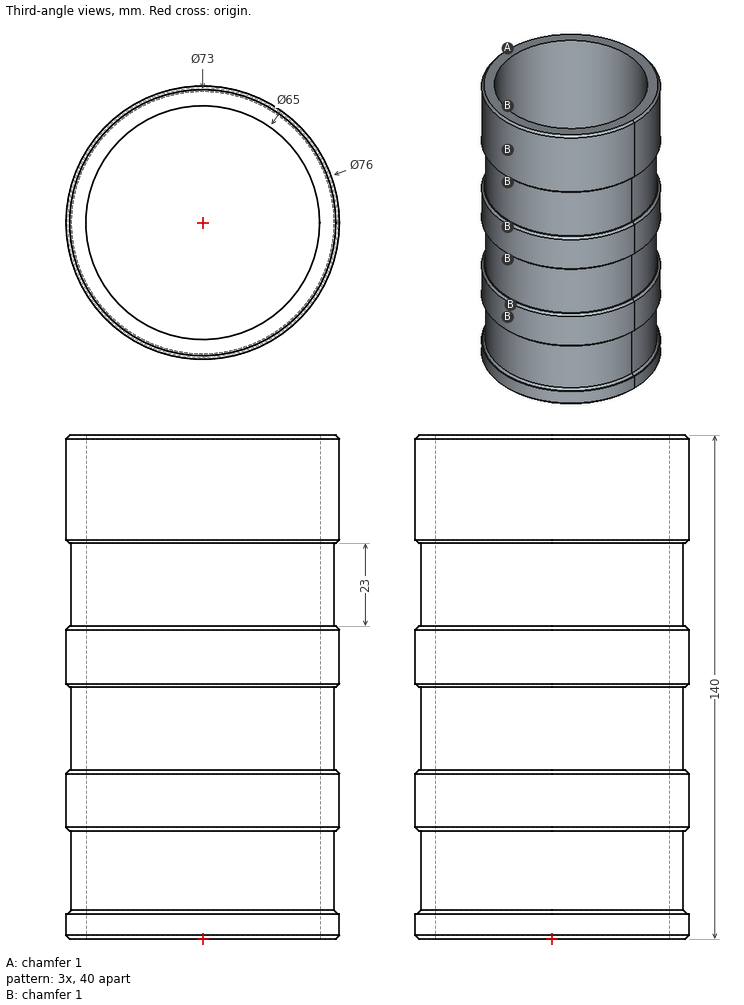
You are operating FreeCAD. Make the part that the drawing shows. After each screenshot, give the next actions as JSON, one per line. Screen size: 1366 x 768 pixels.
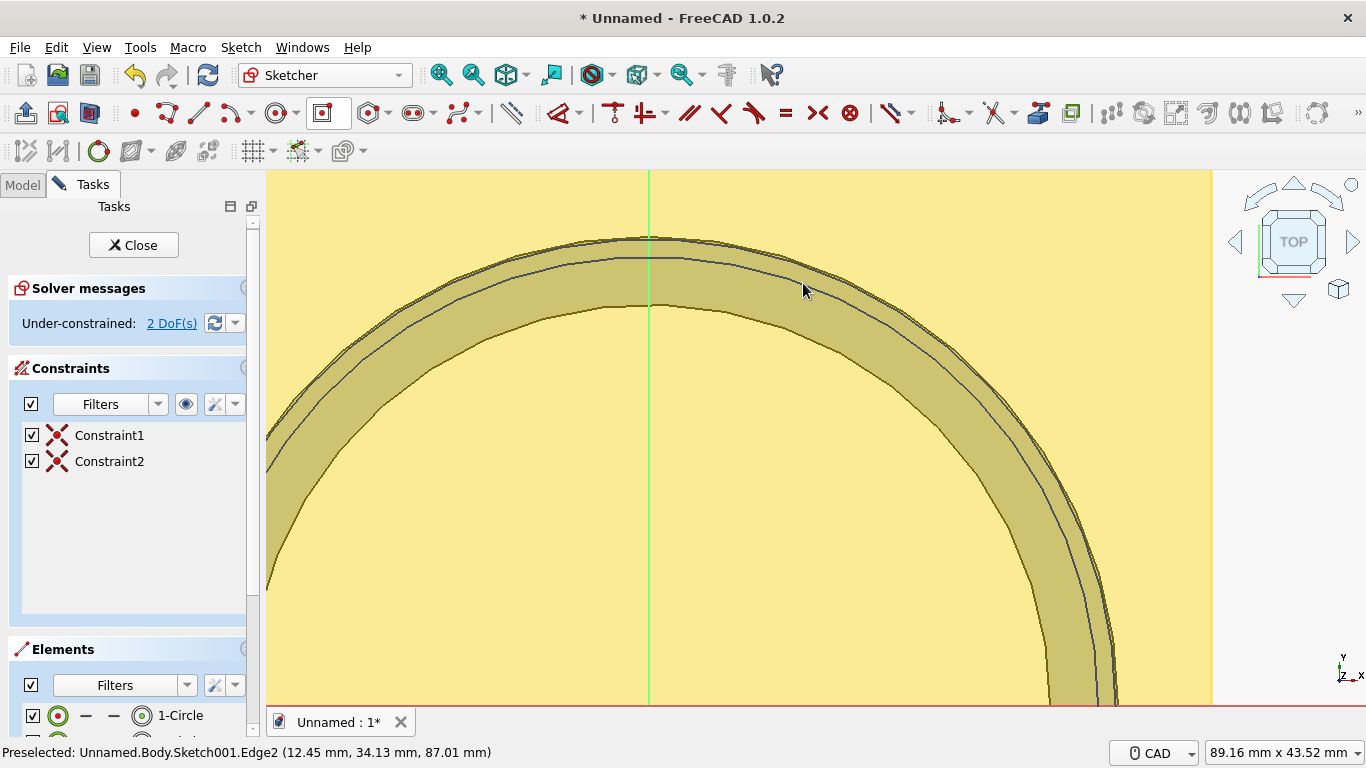
{"action": "left_click", "coordinate": [978, 375]}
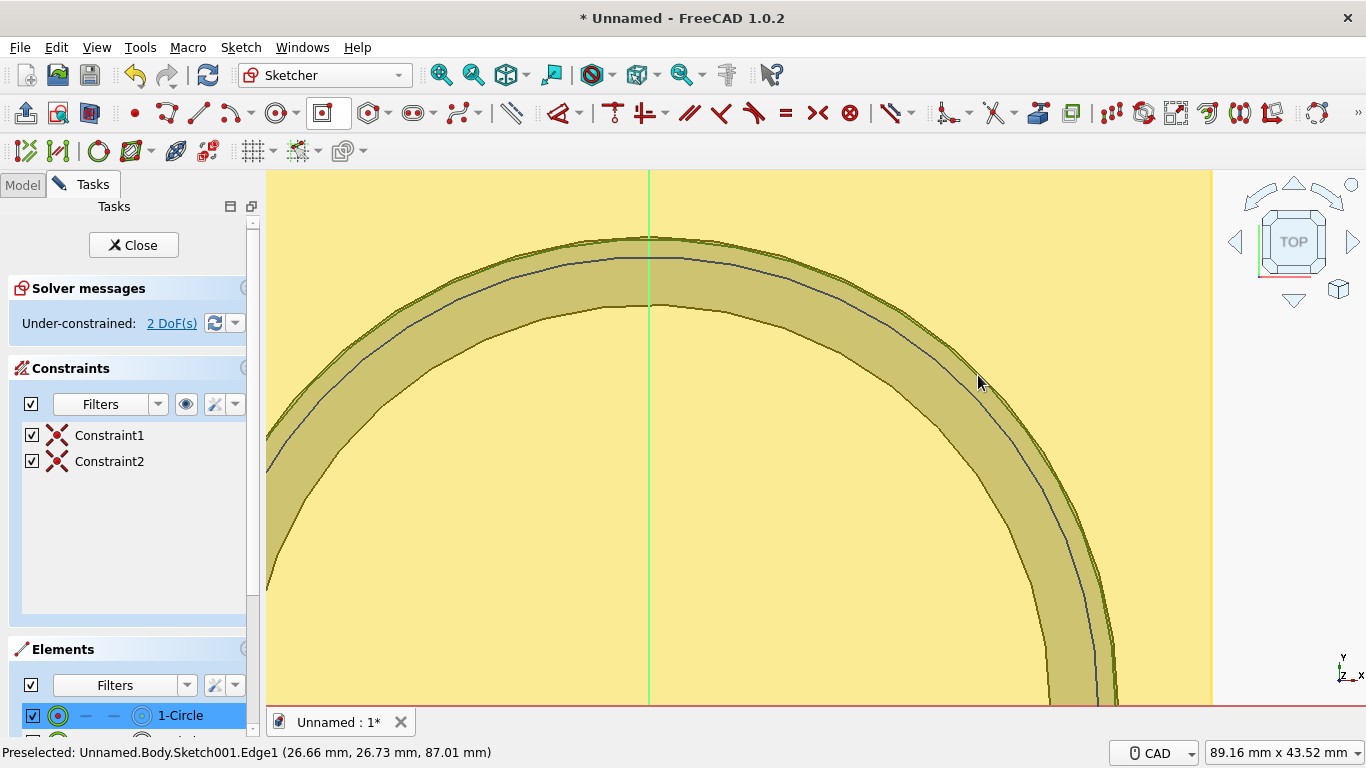
{"action": "left_click", "coordinate": [582, 114]}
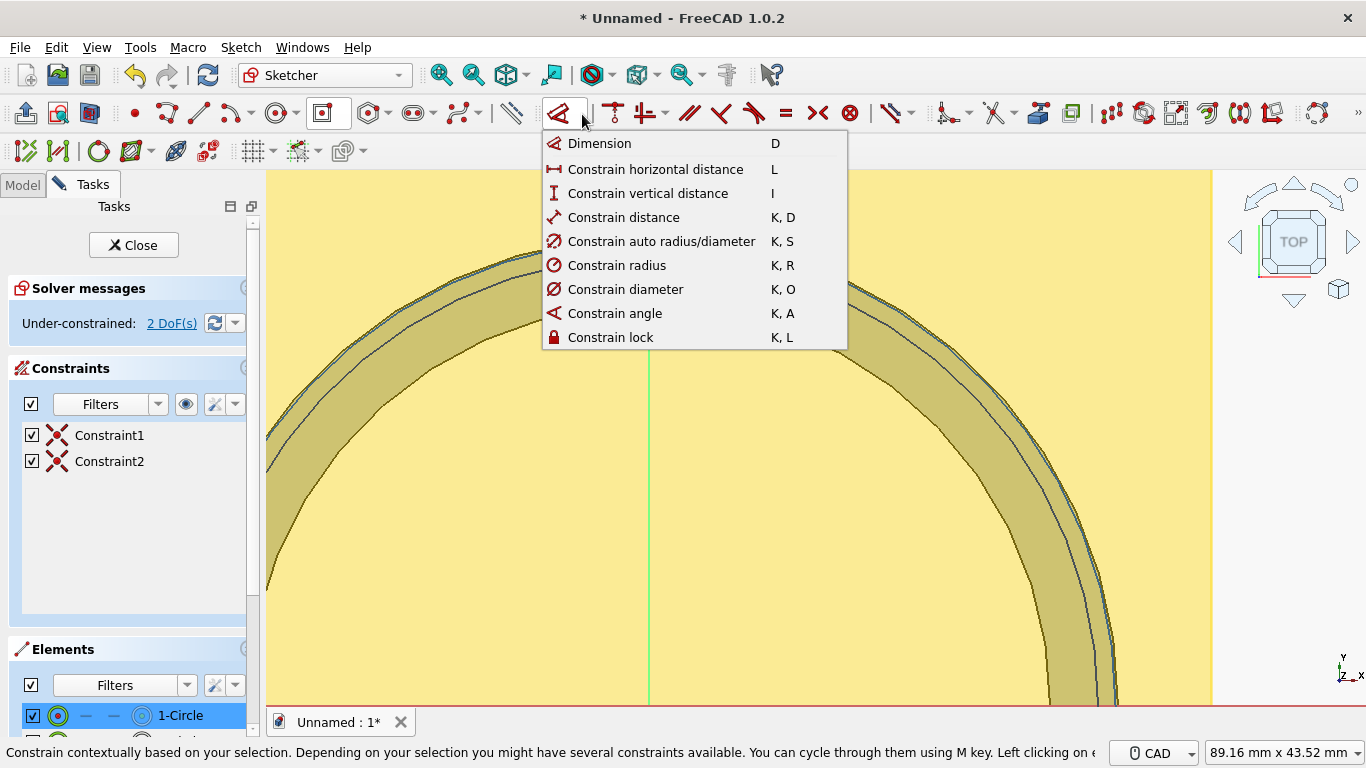
{"action": "left_click", "coordinate": [695, 289]}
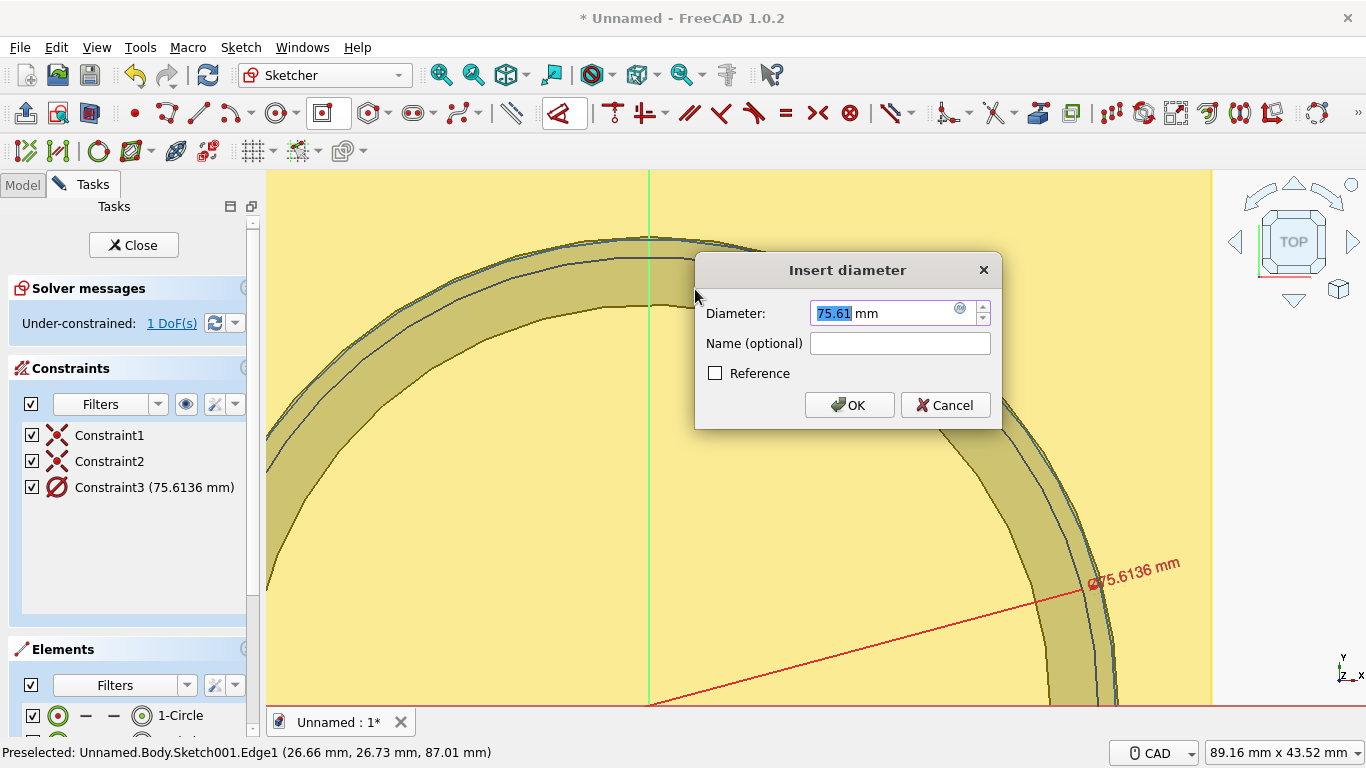
{"action": "type", "text": "76"}
{"action": "key", "text": "Return"}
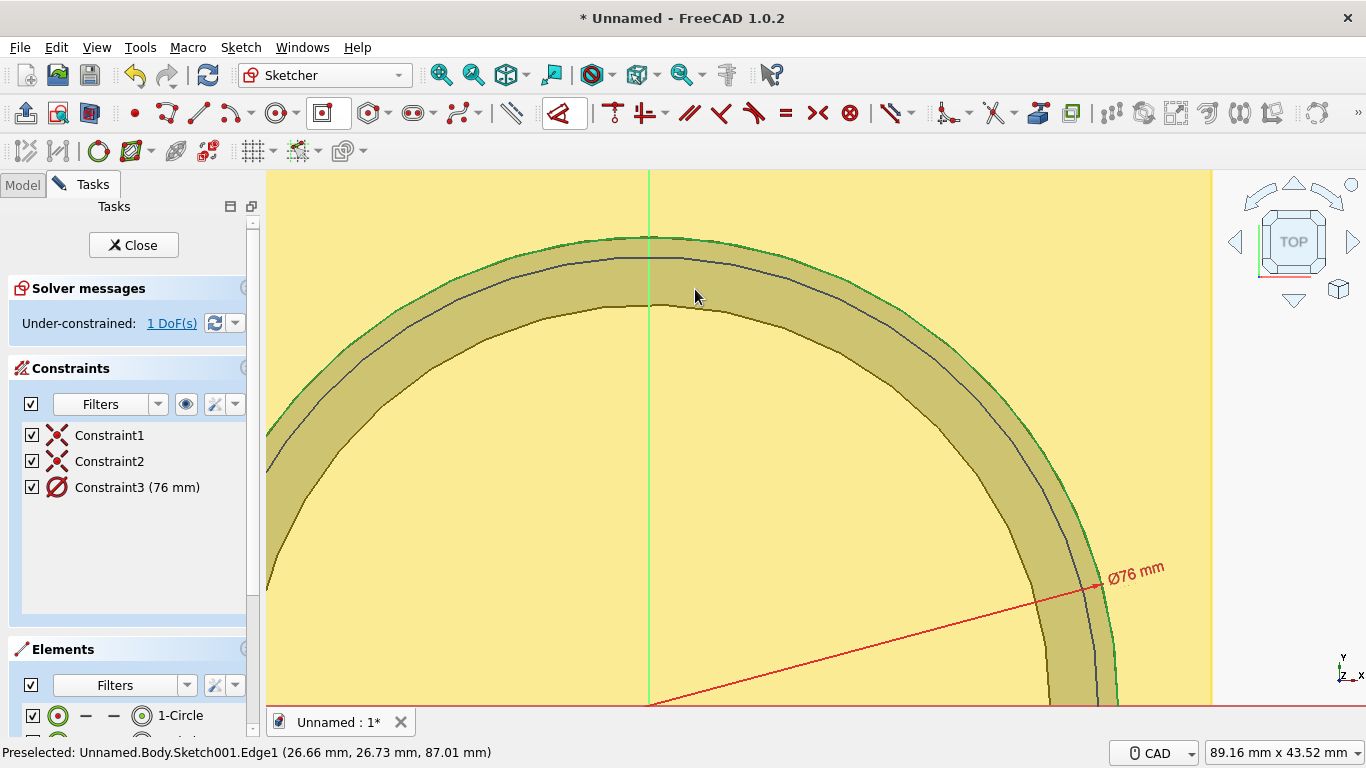
{"action": "left_click", "coordinate": [966, 387]}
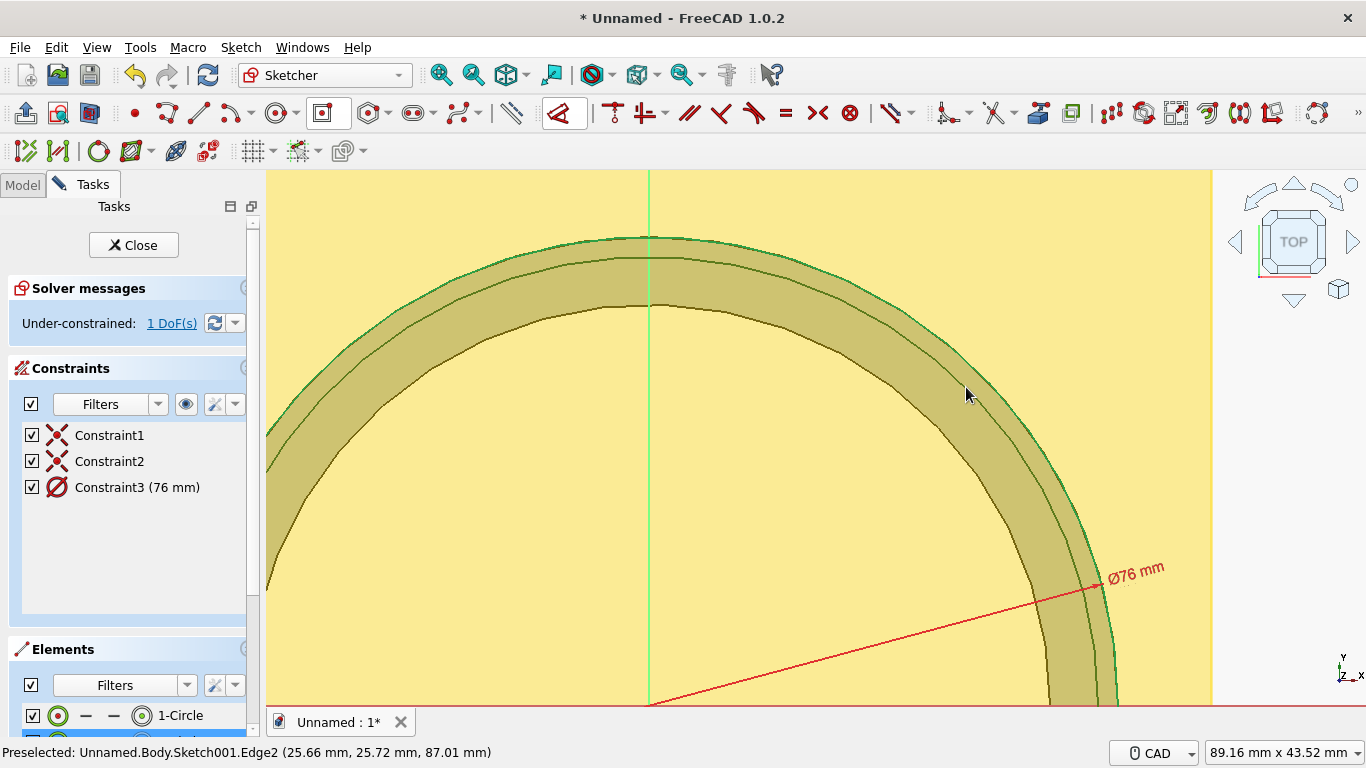
{"action": "key", "text": "k o"}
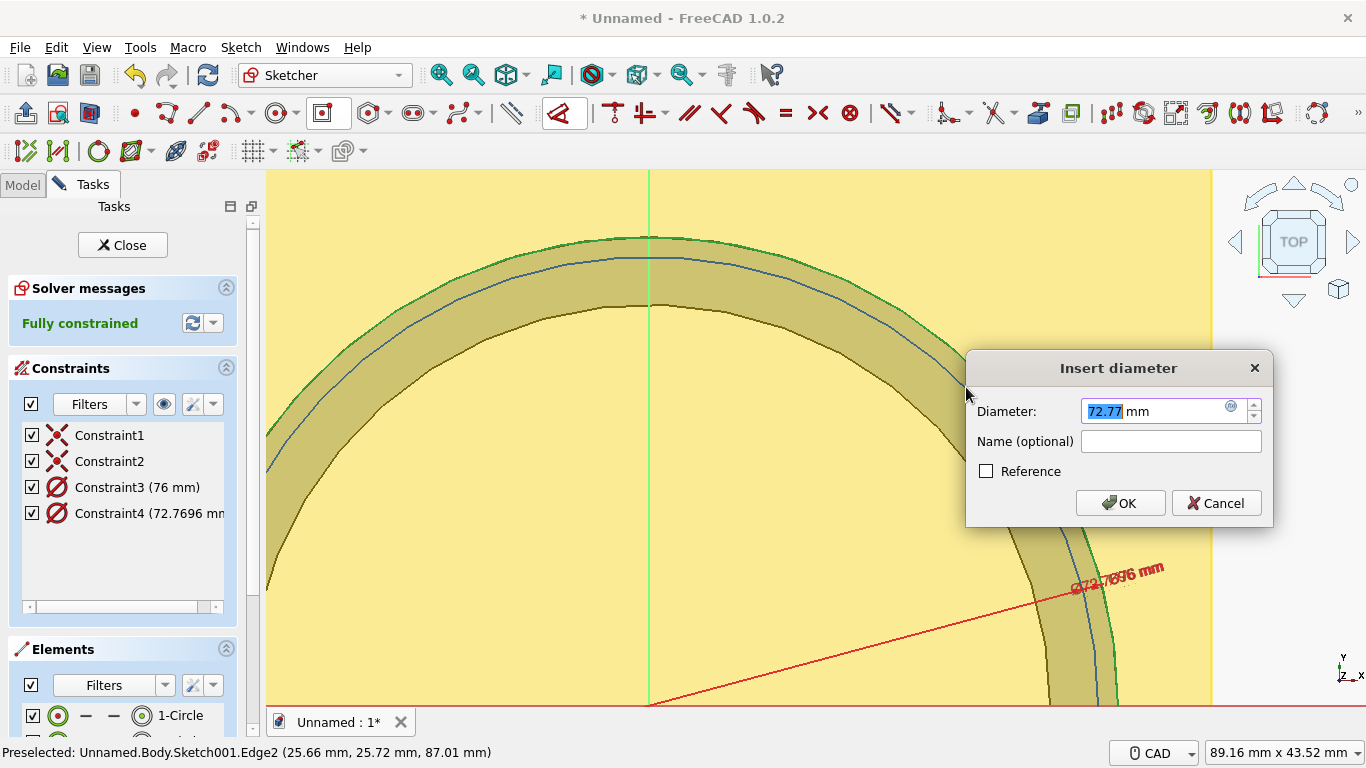
{"action": "type", "text": "73"}
{"action": "key", "text": "Return"}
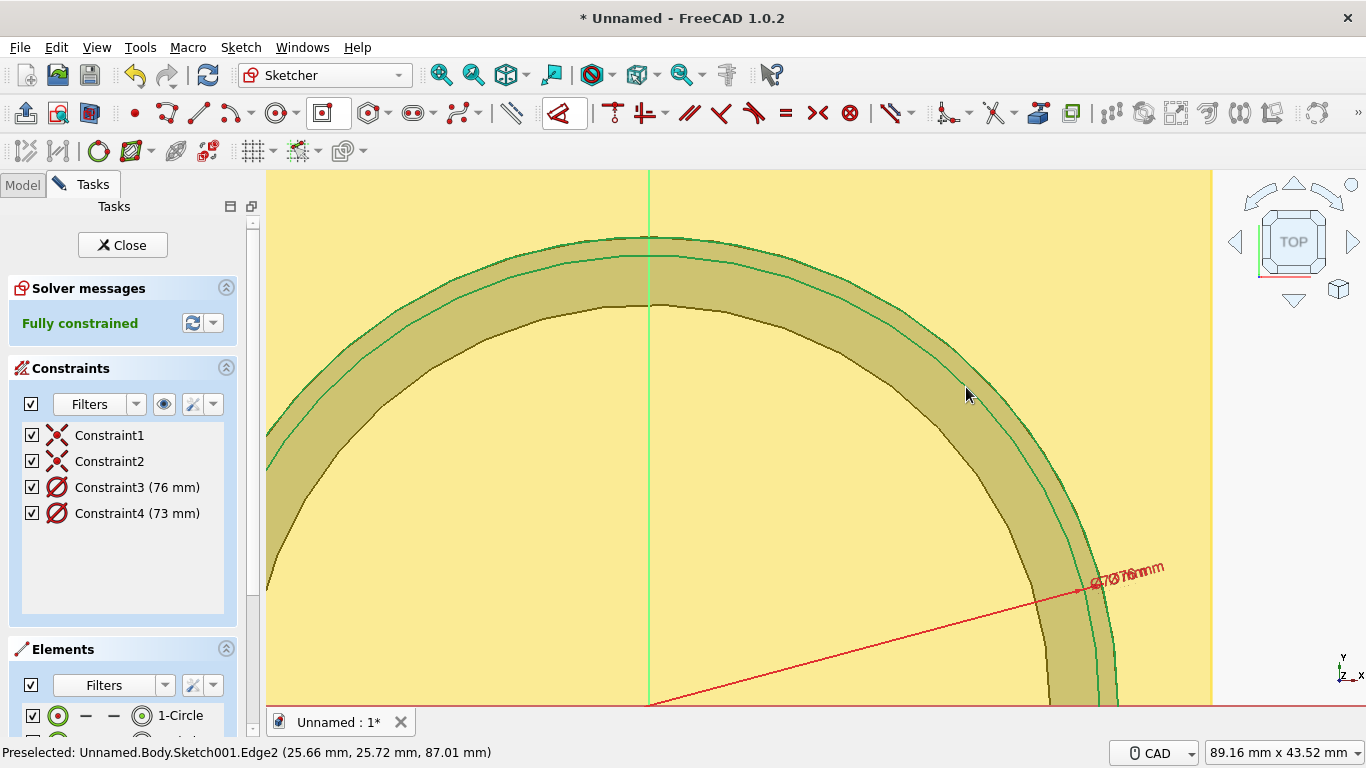
{"action": "left_click", "coordinate": [123, 245]}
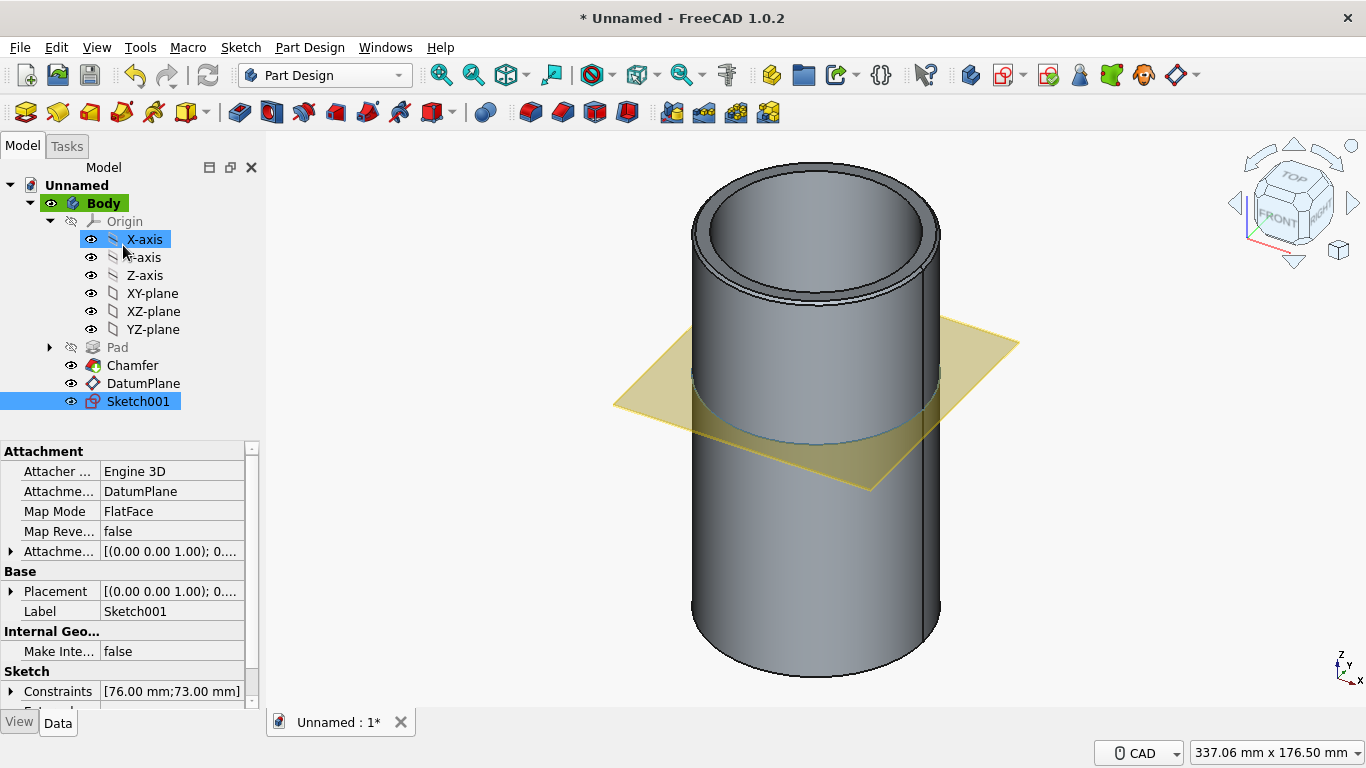
{"action": "left_click", "coordinate": [240, 112]}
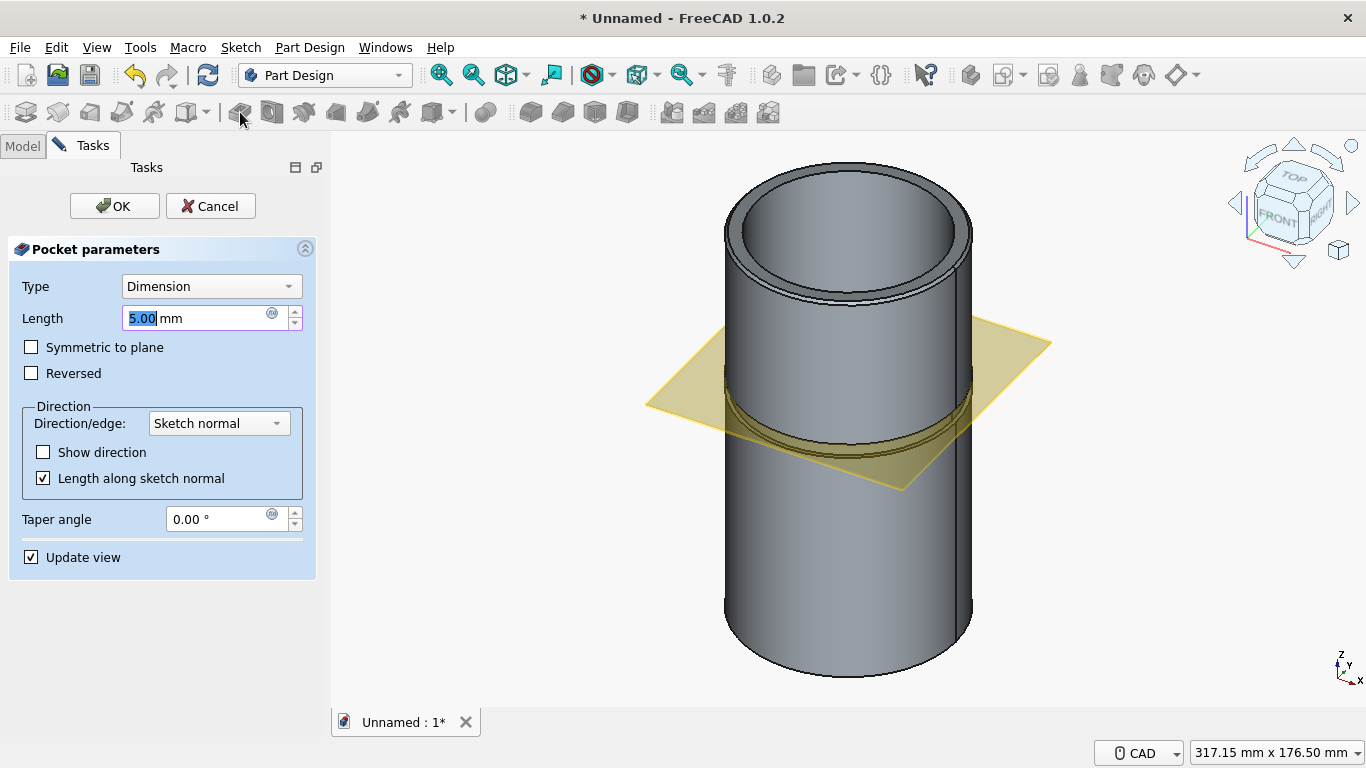
{"action": "type", "text": "23"}
{"action": "key", "text": "Tab"}